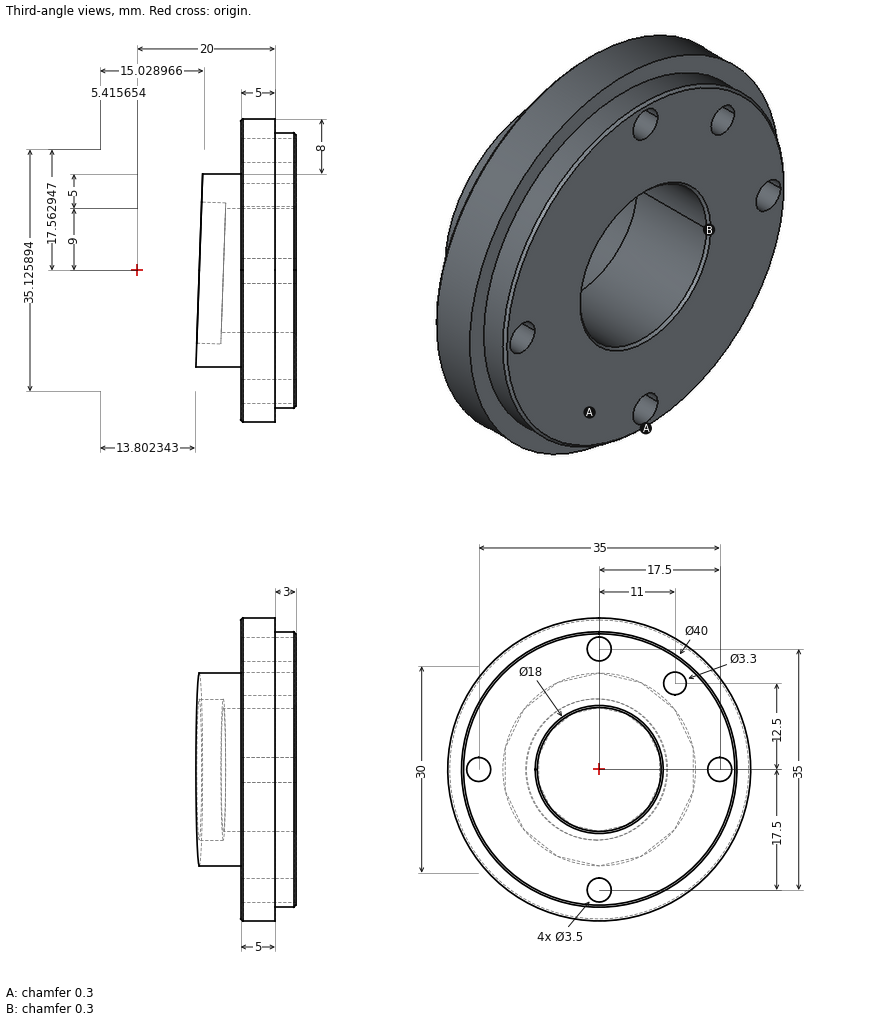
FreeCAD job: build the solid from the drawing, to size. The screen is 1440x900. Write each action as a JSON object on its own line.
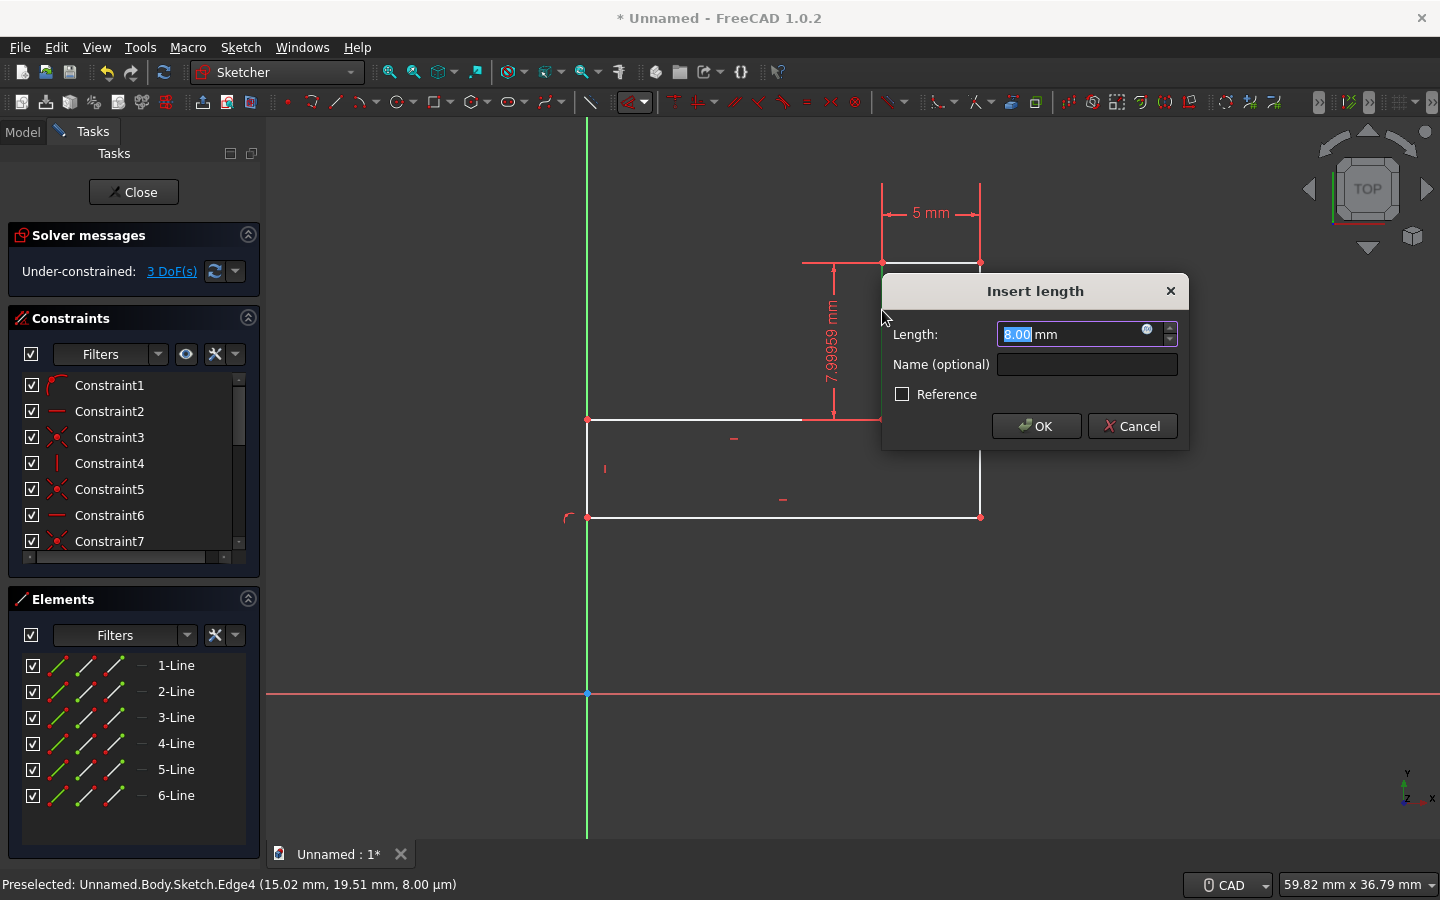
{"action": "type", "text": "8"}
{"action": "key", "text": "Return"}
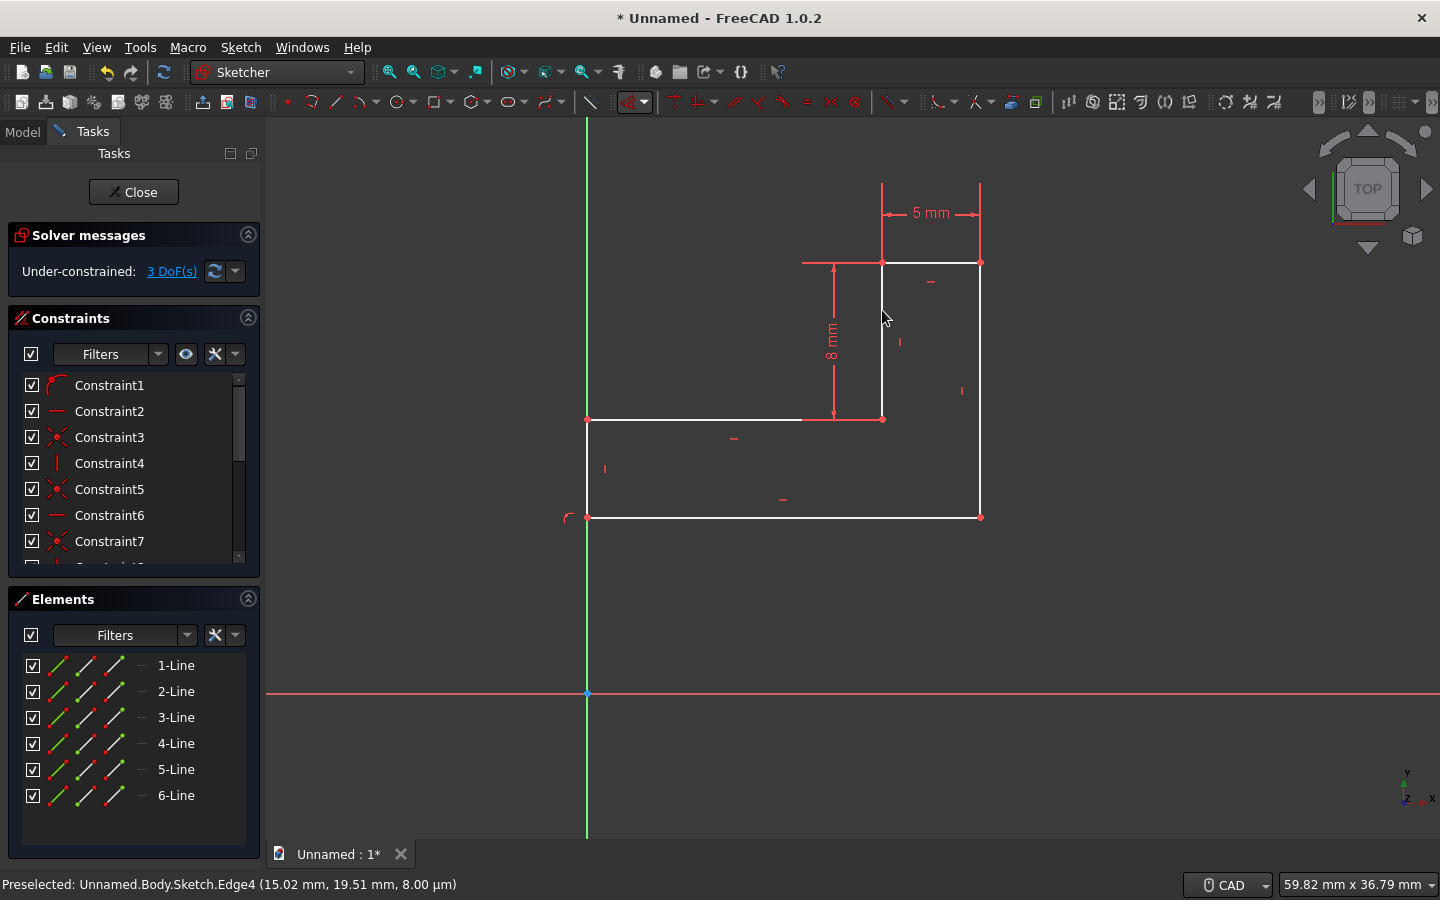
{"action": "left_click", "coordinate": [587, 449]}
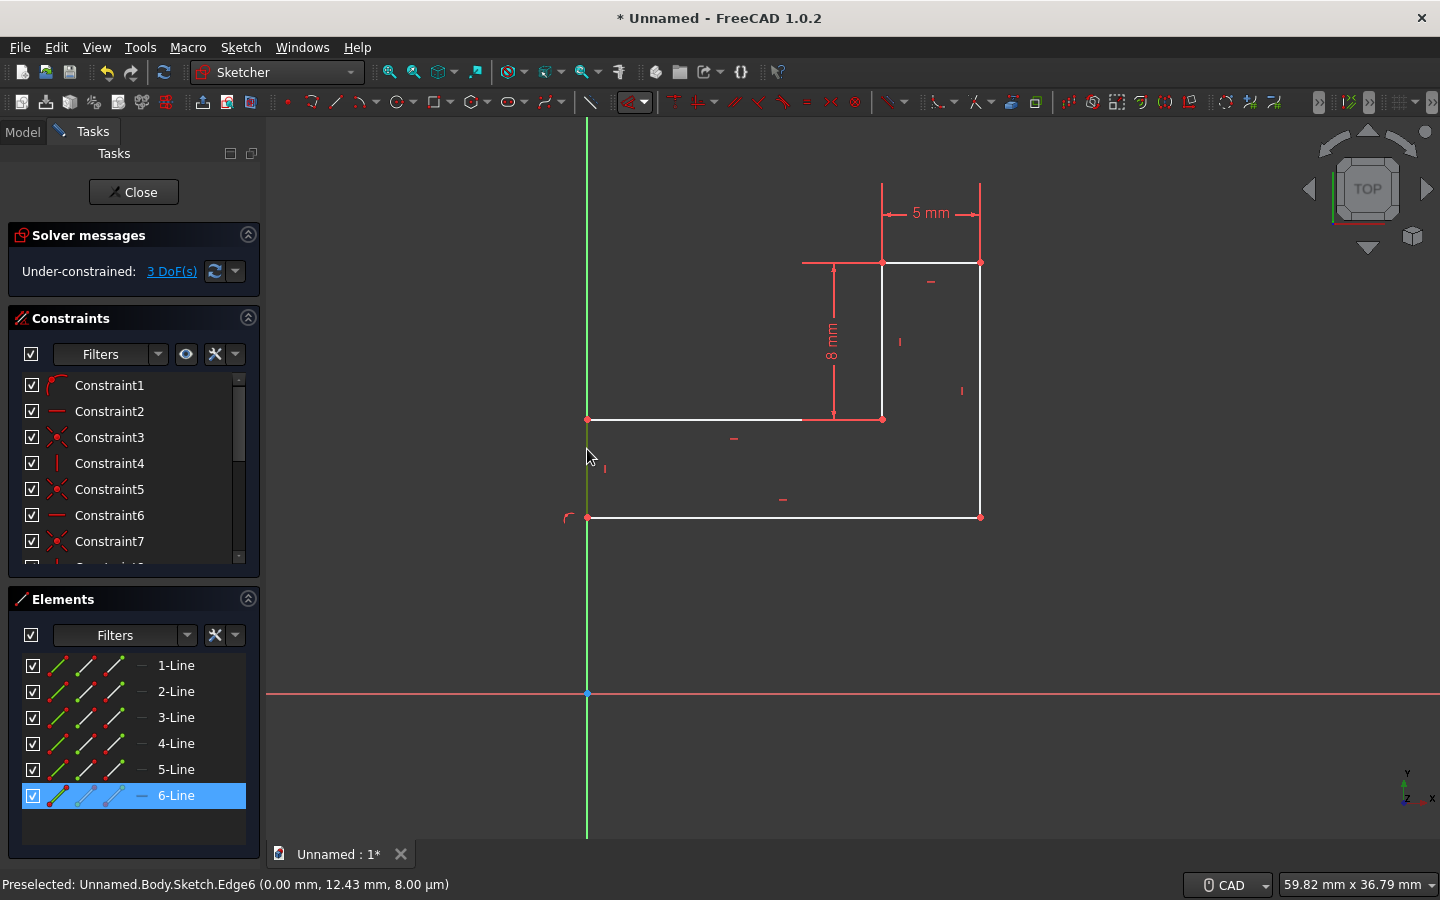
{"action": "left_click", "coordinate": [646, 102]}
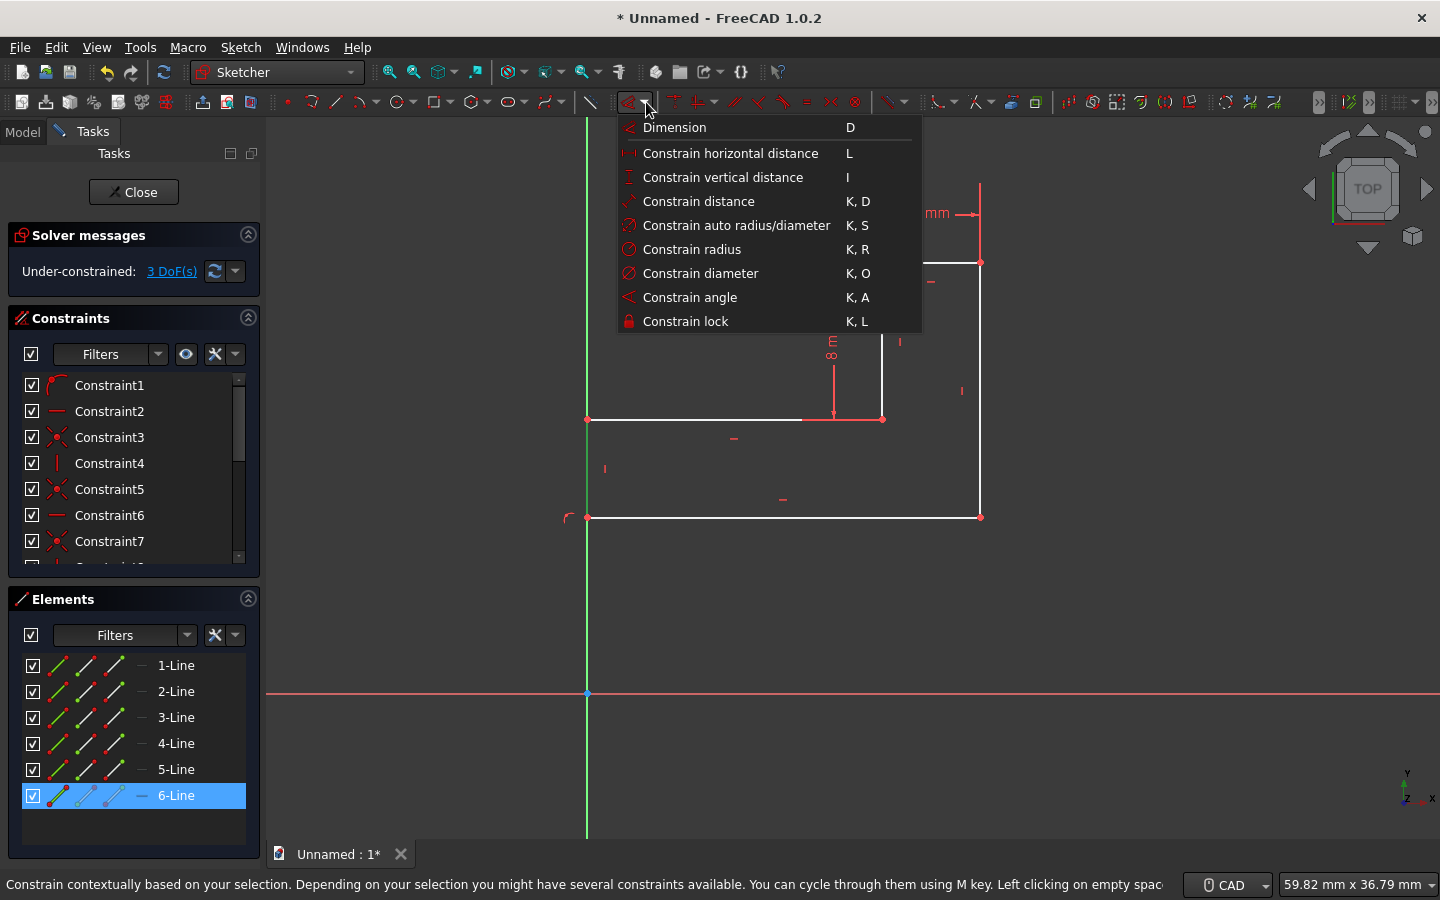
{"action": "left_click", "coordinate": [770, 177]}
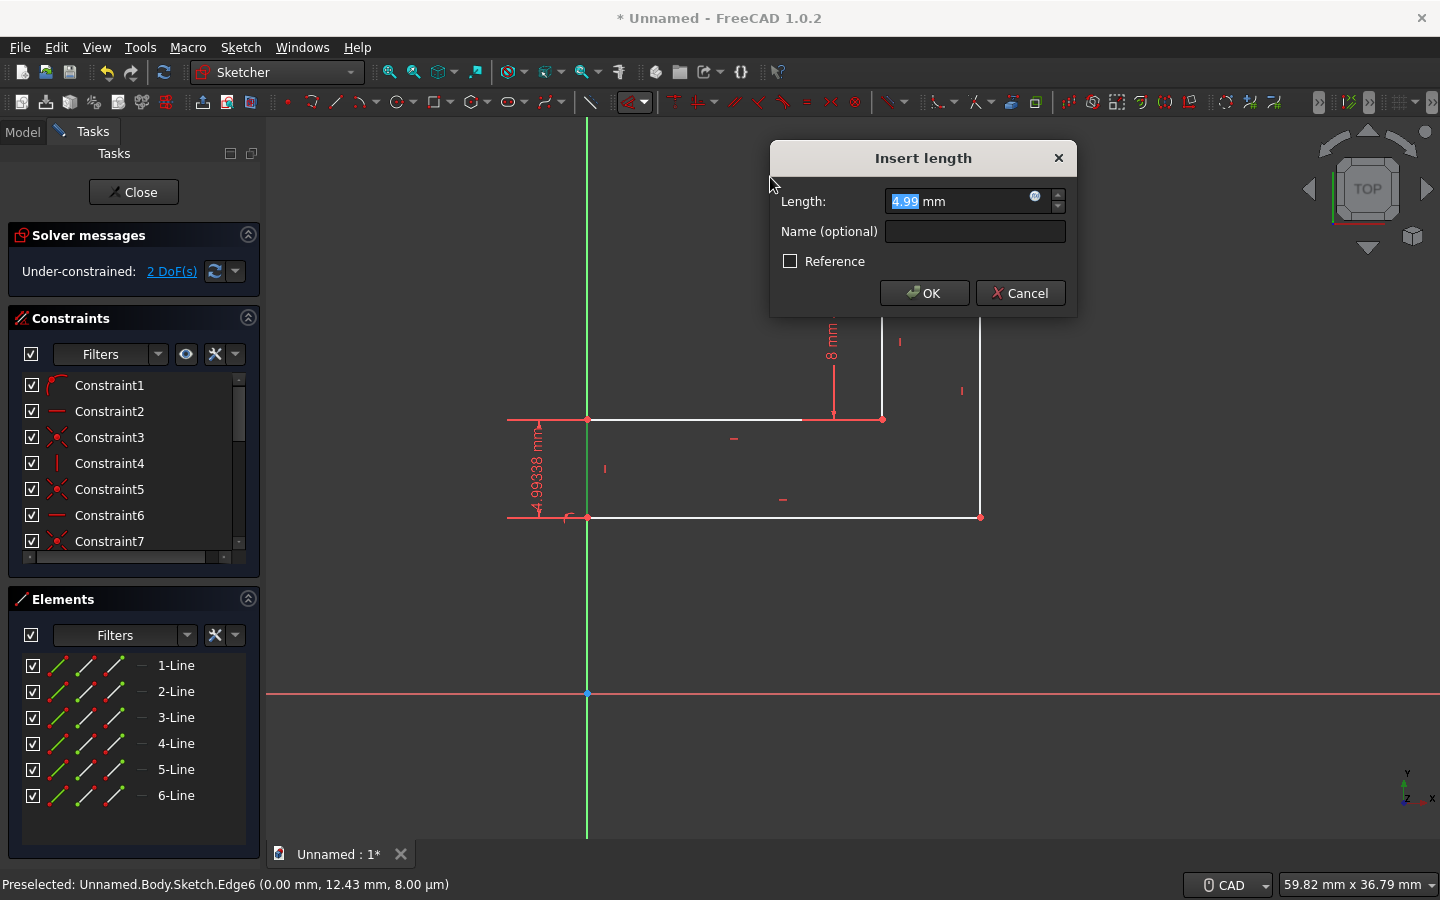
{"action": "type", "text": "5"}
{"action": "key", "text": "Return"}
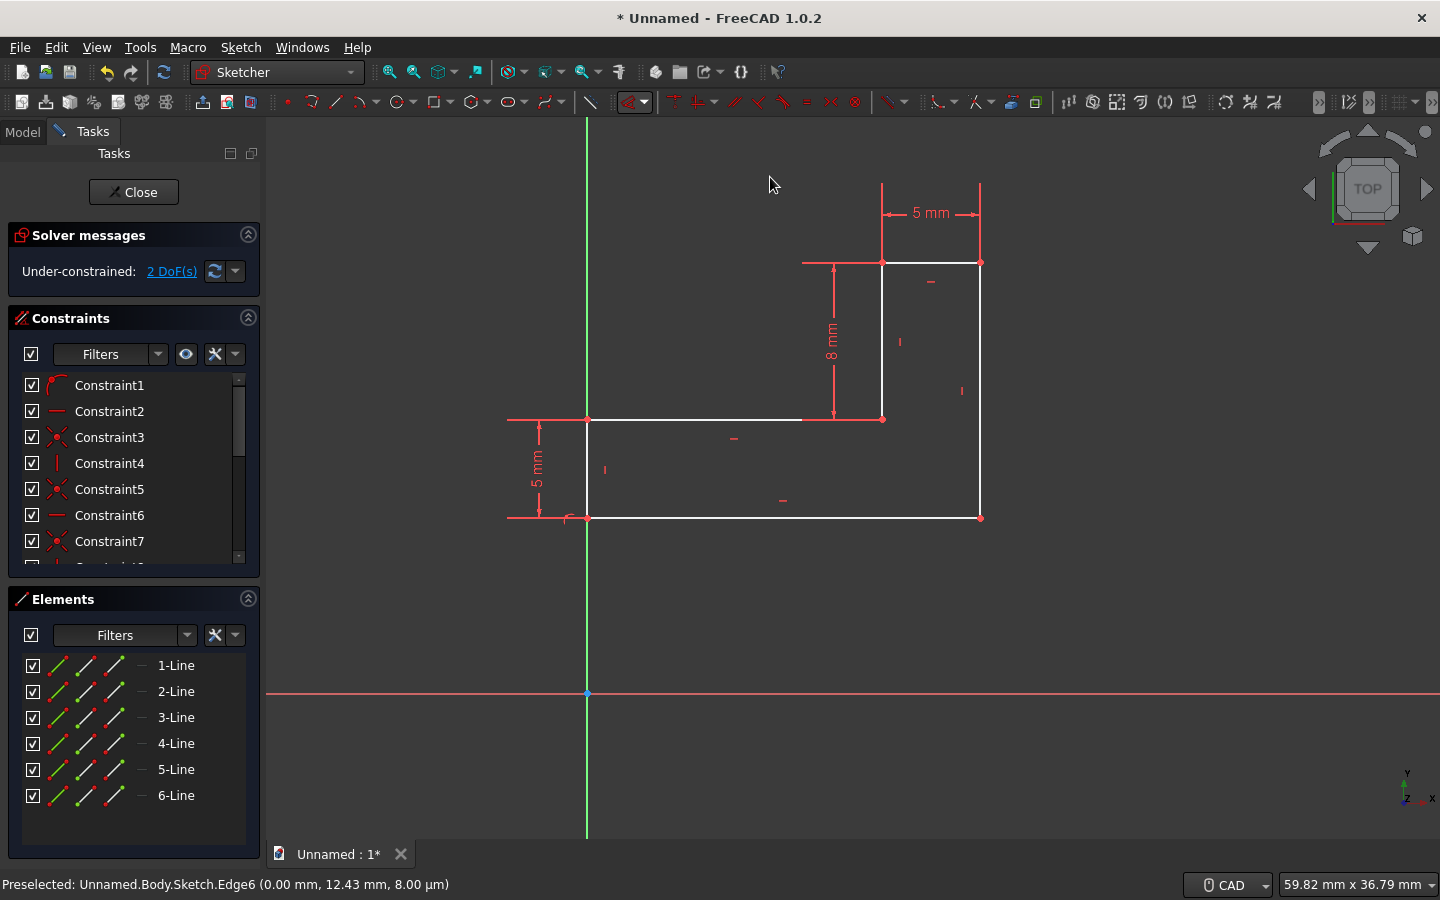
{"action": "left_click", "coordinate": [705, 518]}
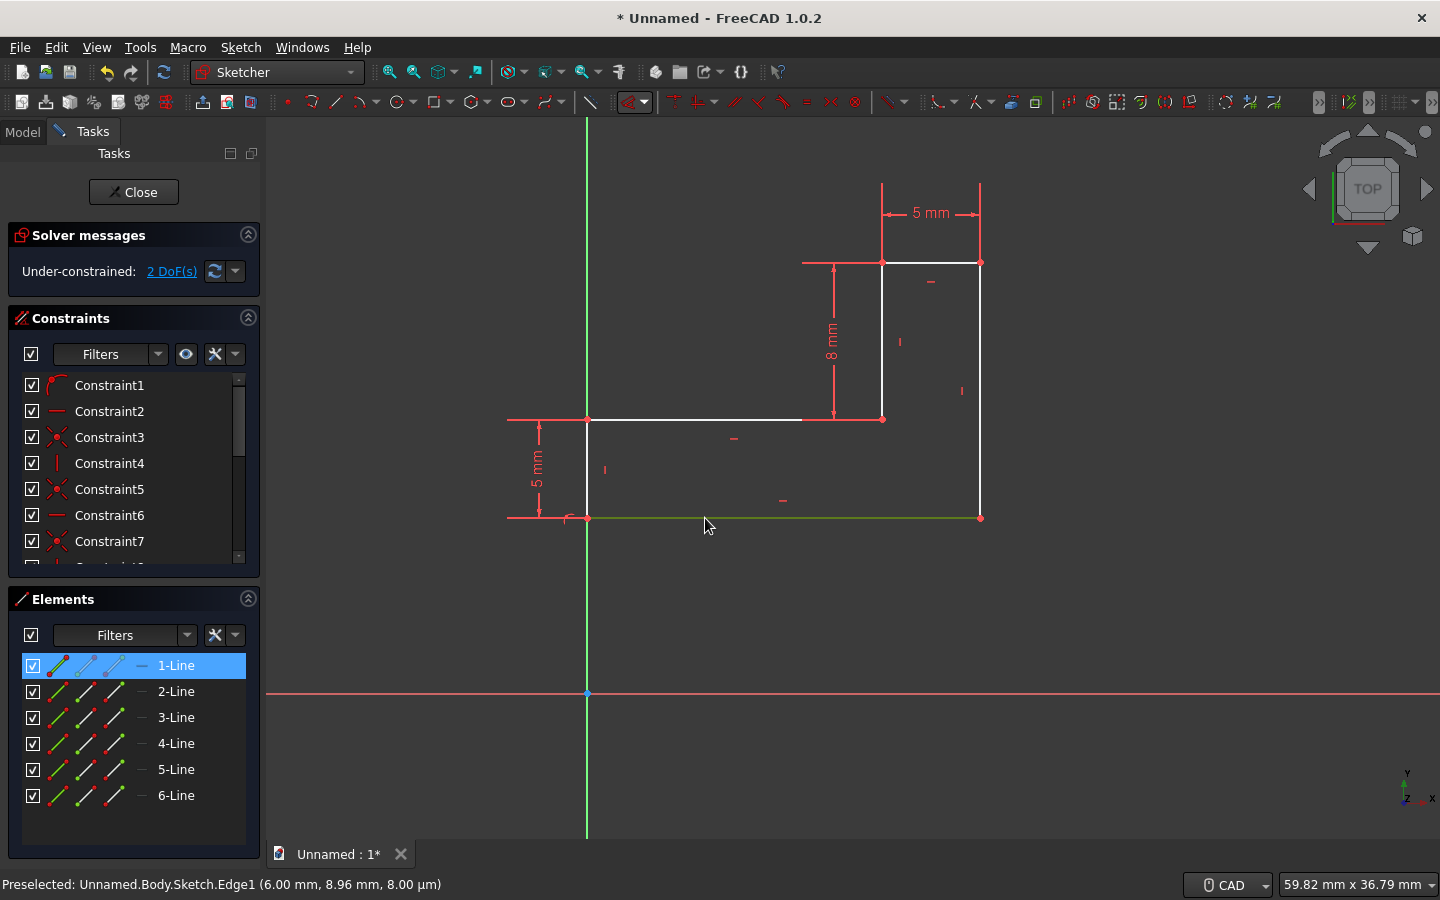
{"action": "key", "text": "l"}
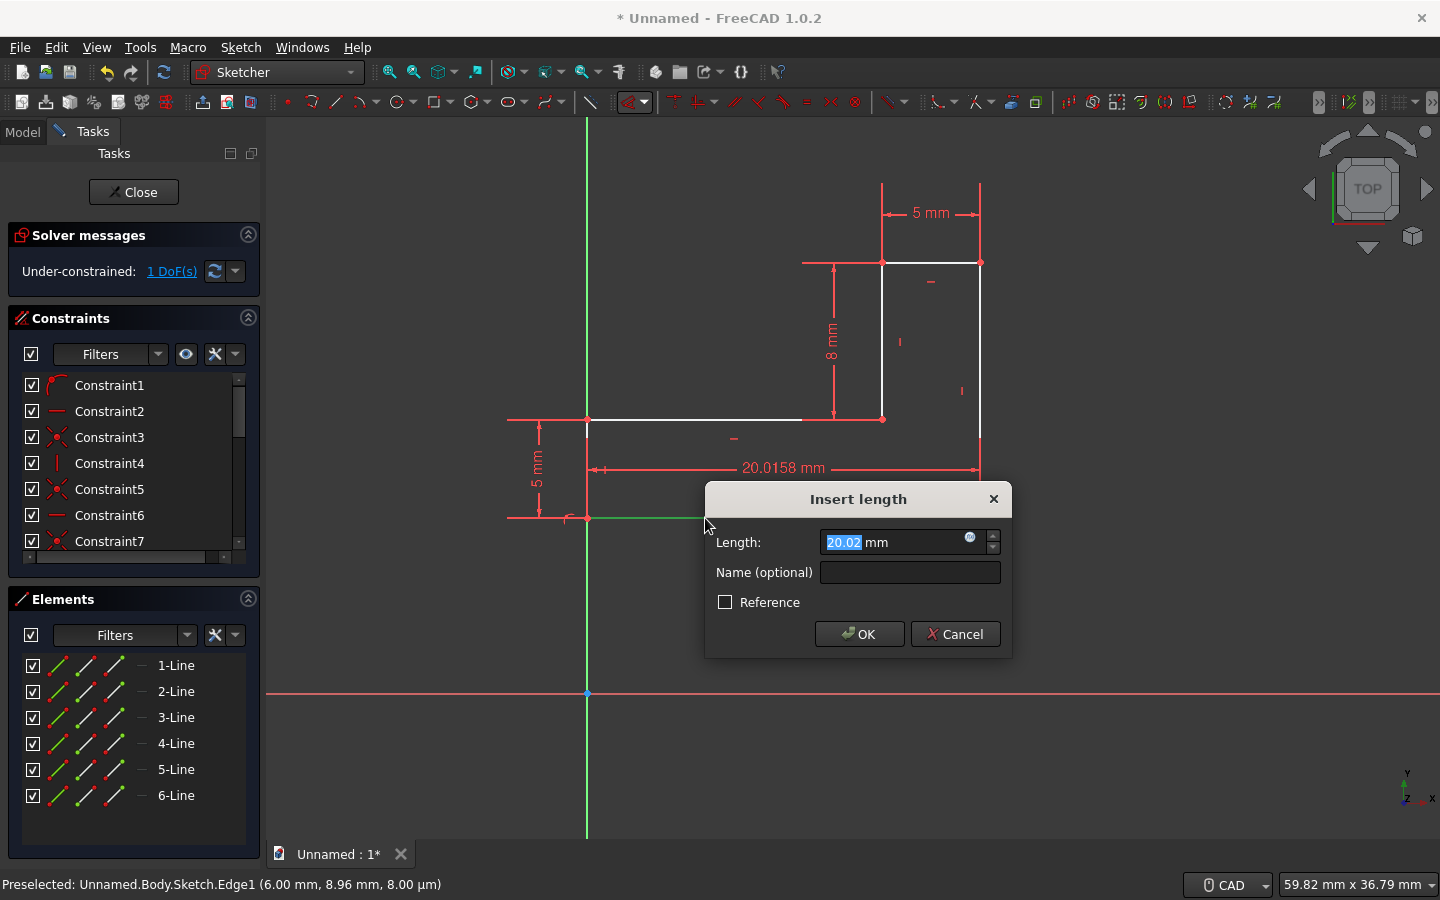
{"action": "type", "text": "20"}
{"action": "key", "text": "Return"}